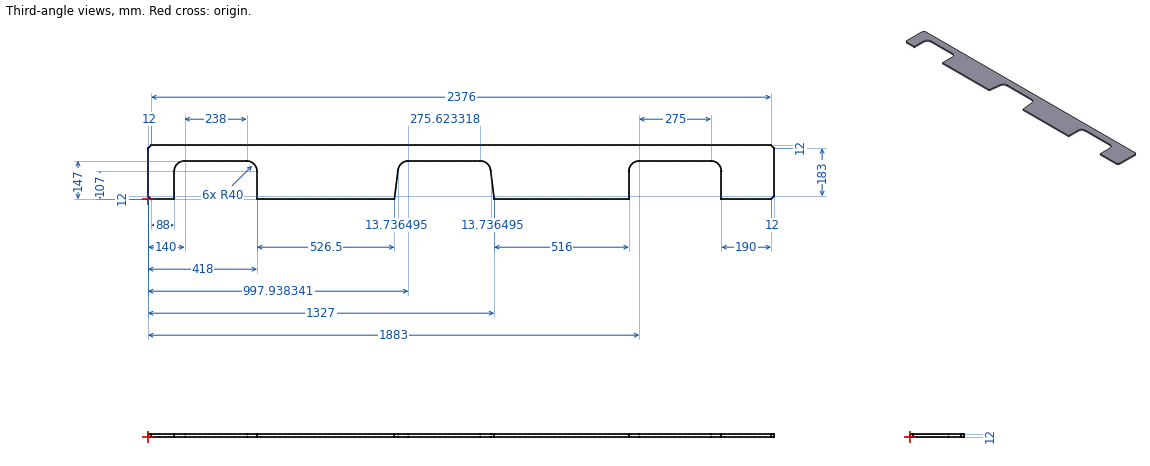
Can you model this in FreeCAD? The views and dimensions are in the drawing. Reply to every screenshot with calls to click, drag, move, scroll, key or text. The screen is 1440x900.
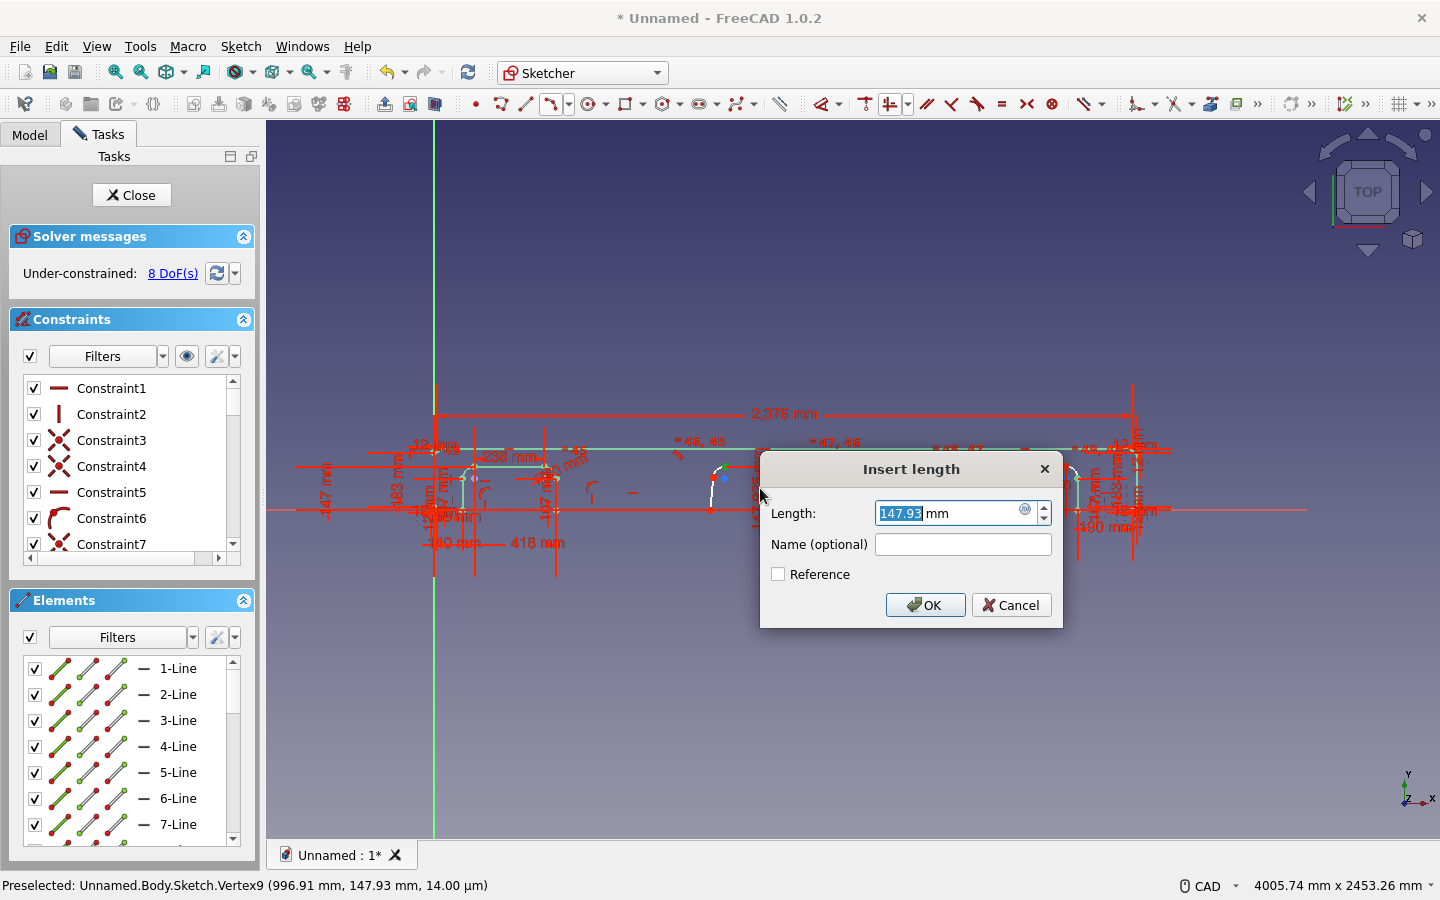
text(147)
key(Return)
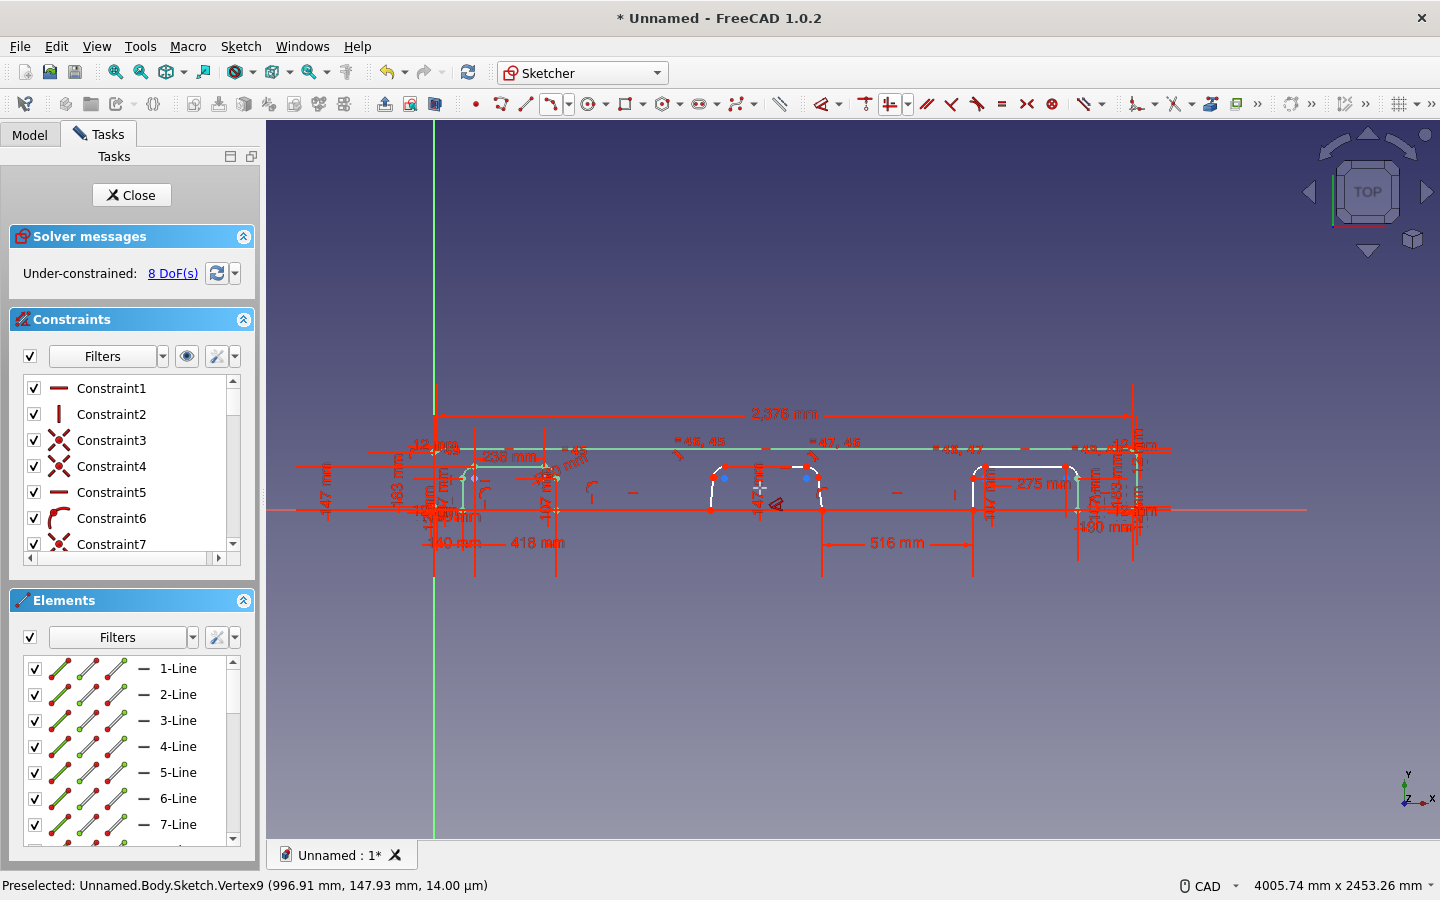
click(985, 467)
click(400, 498)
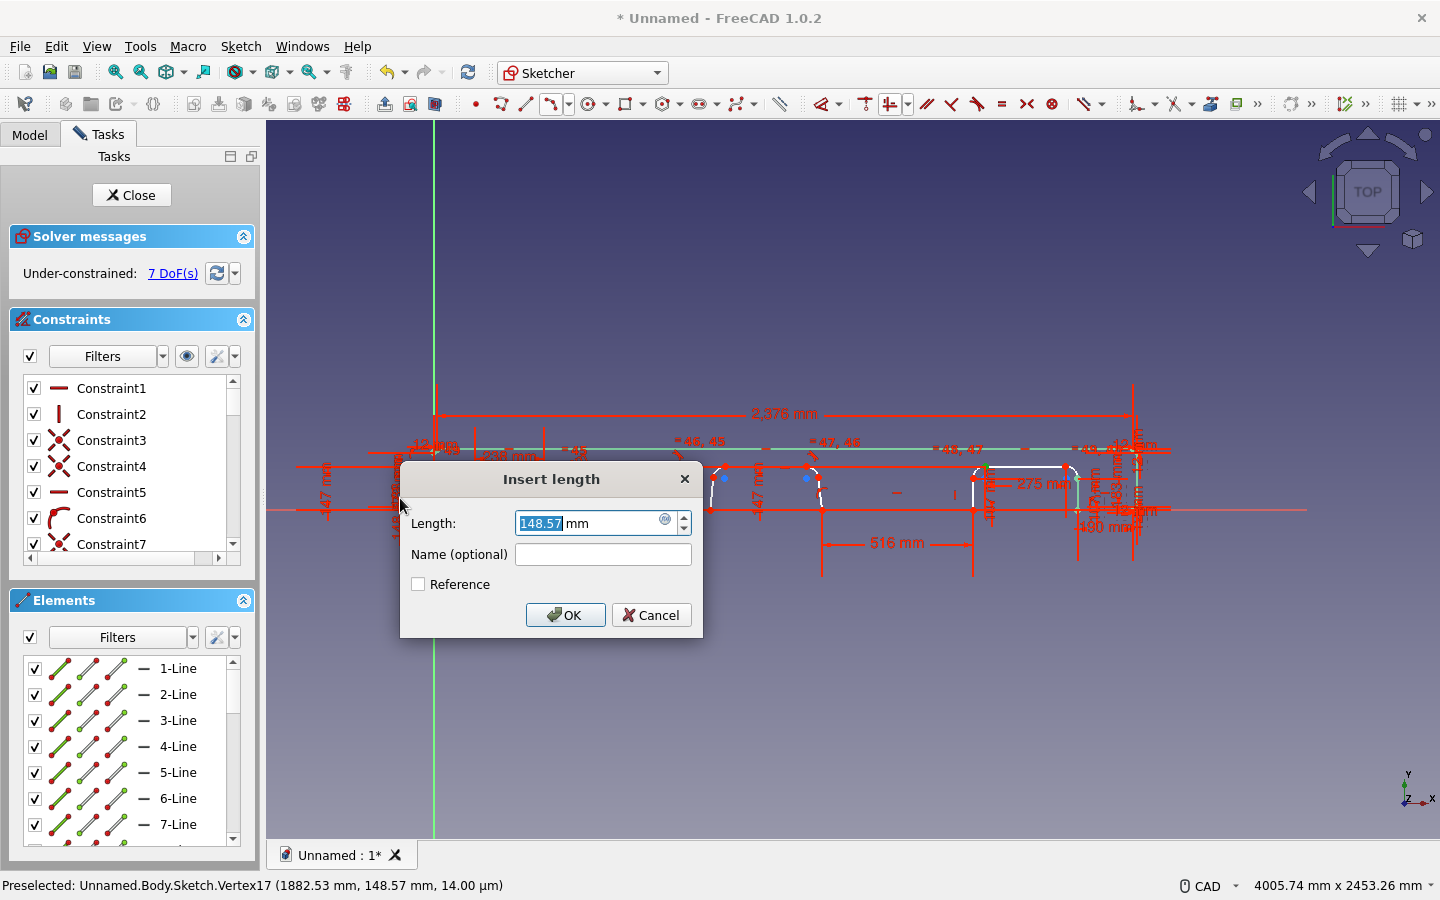
text(147)
key(Return)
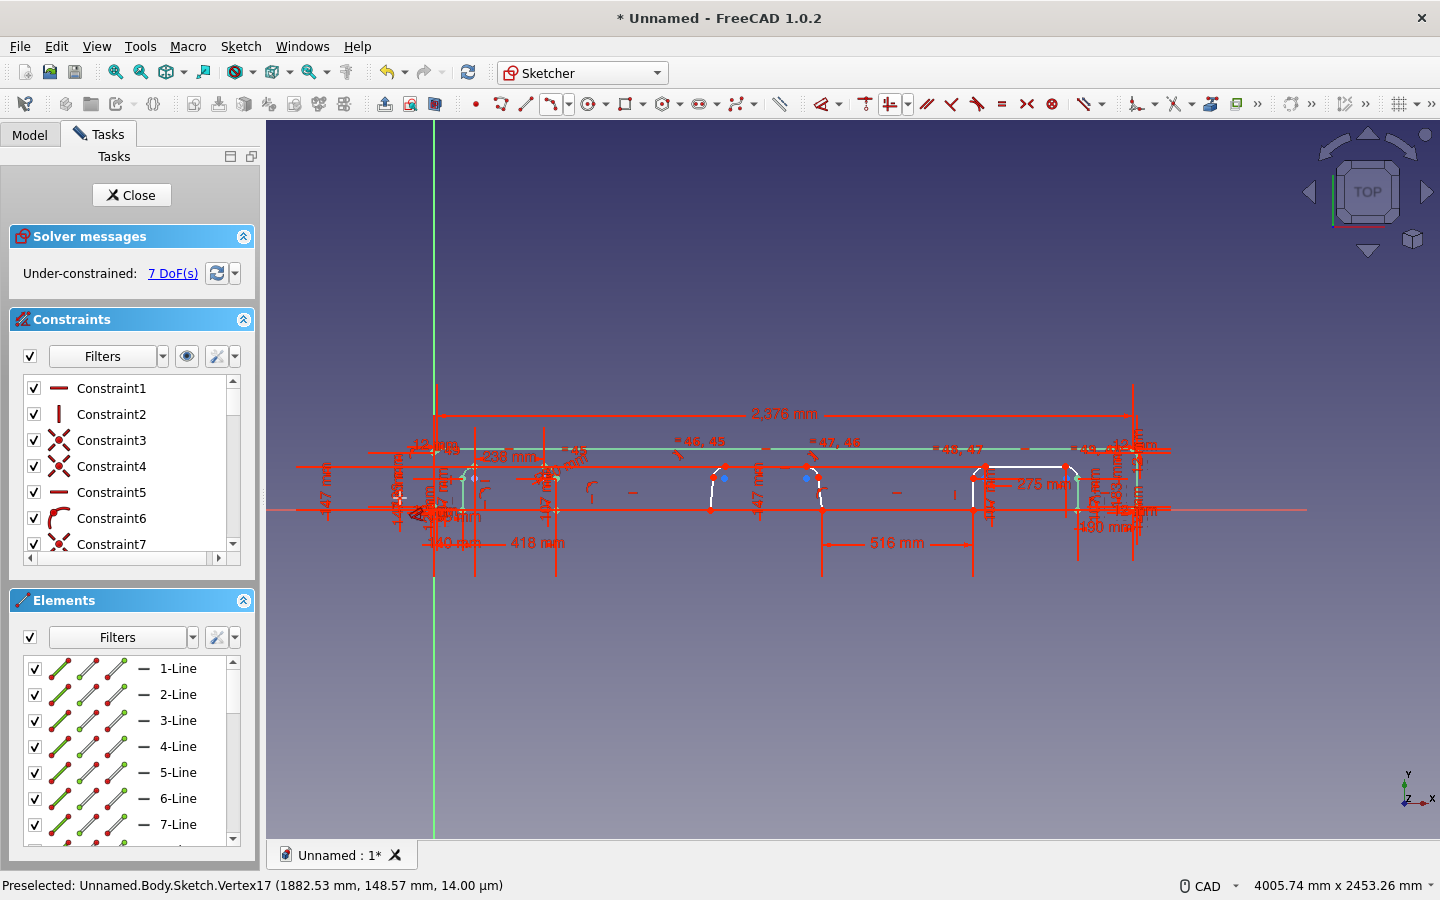
click(602, 510)
click(633, 544)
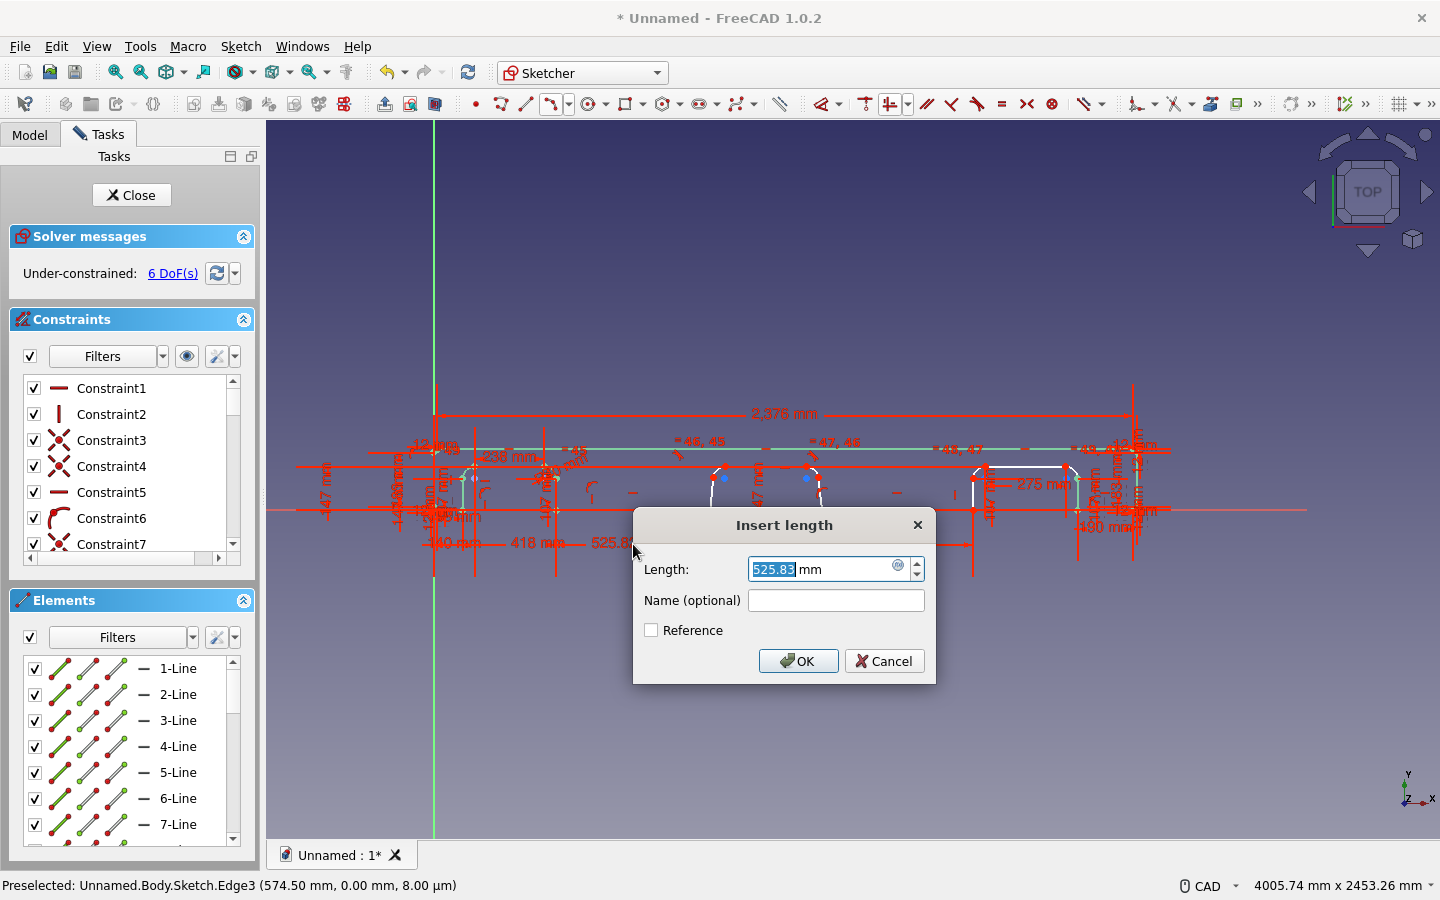
text(526.5)
key(Return)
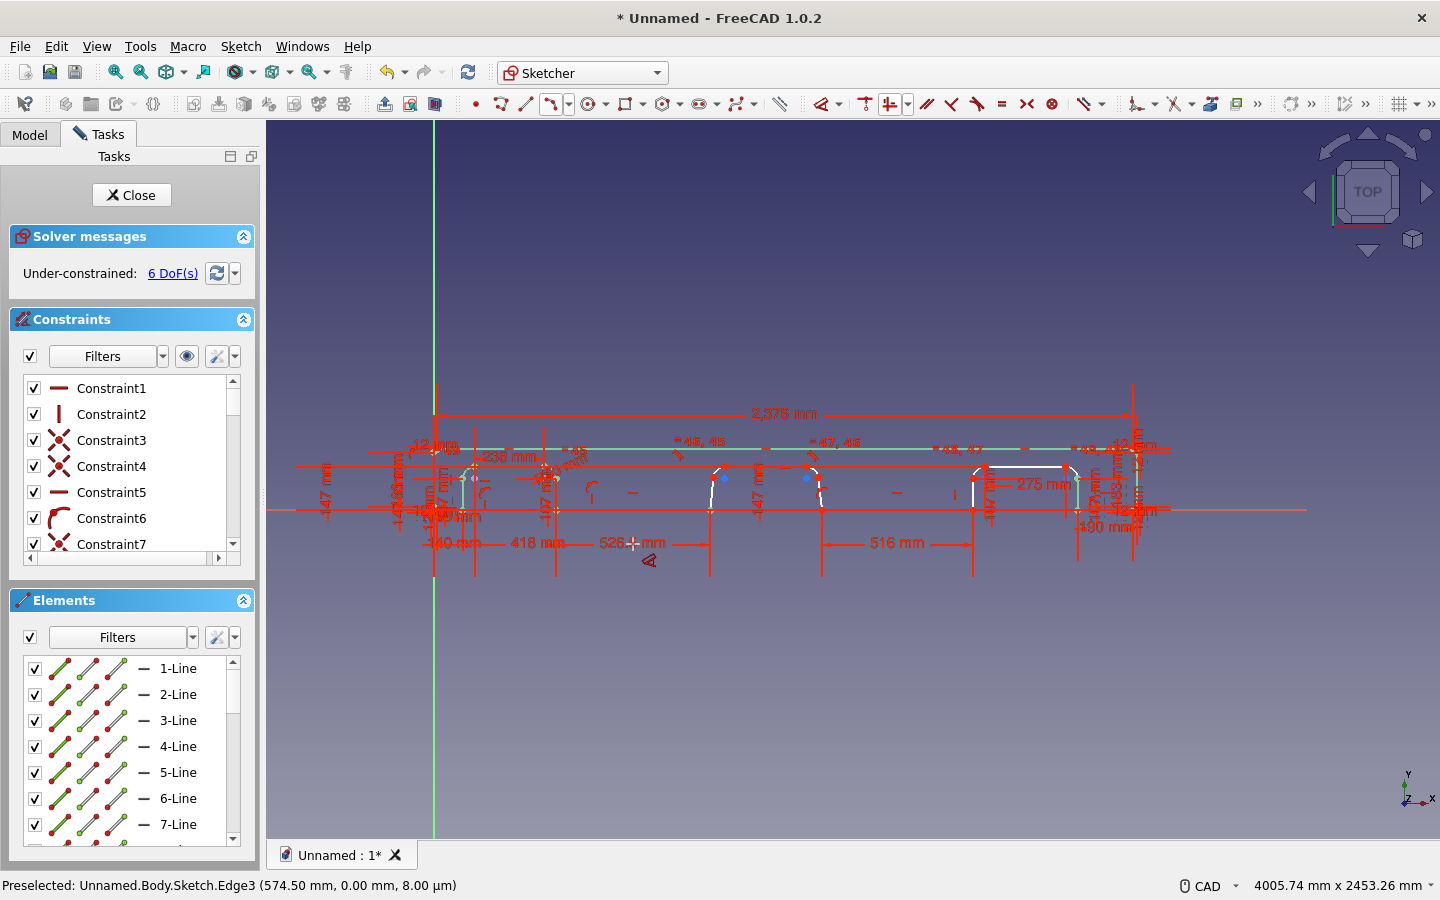
click(822, 510)
click(717, 544)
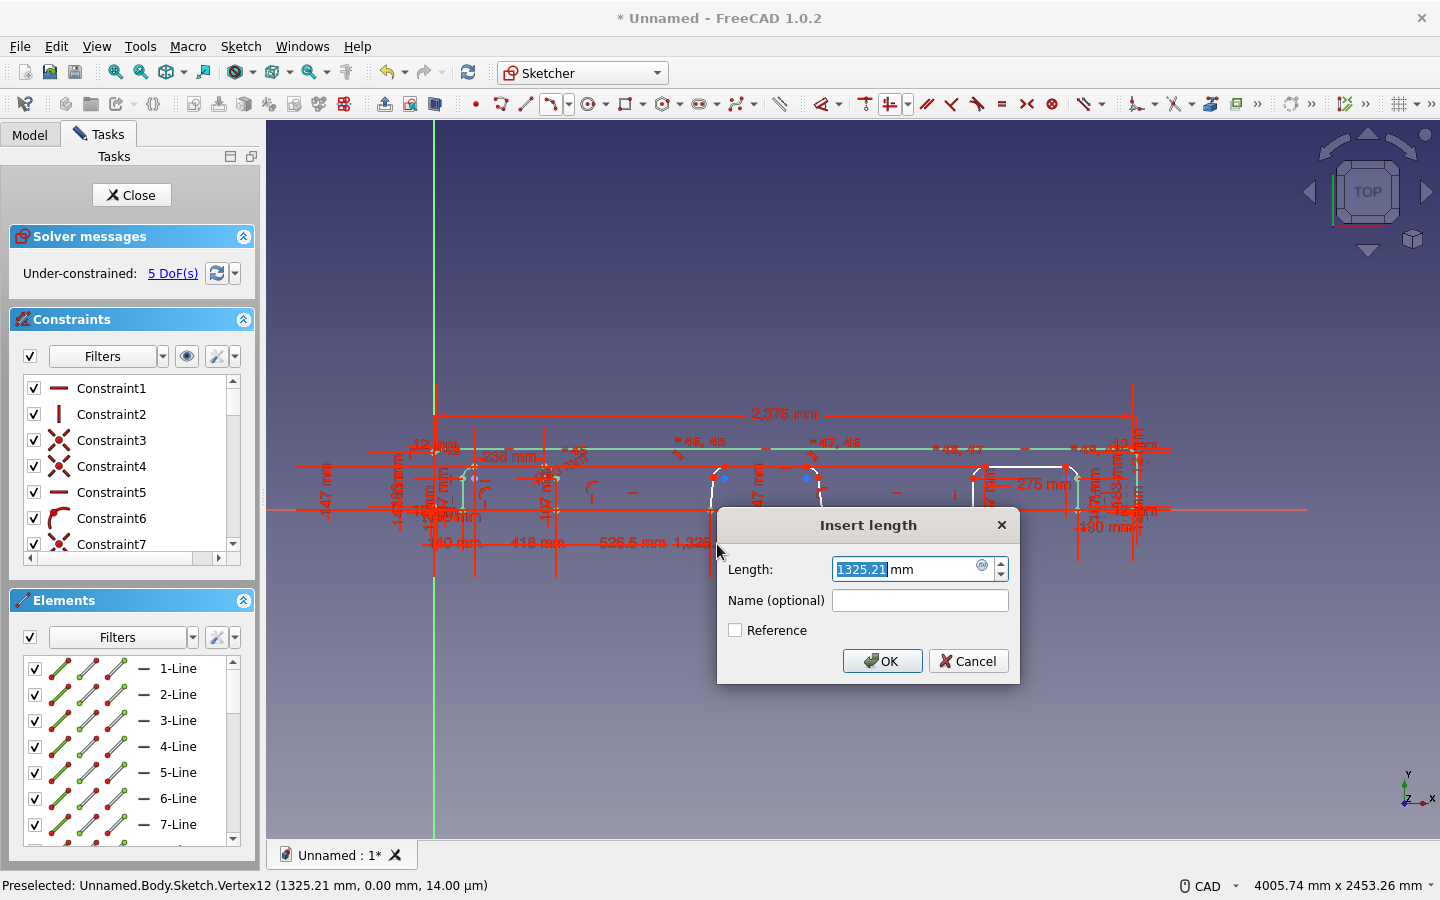
text(1327)
key(Return)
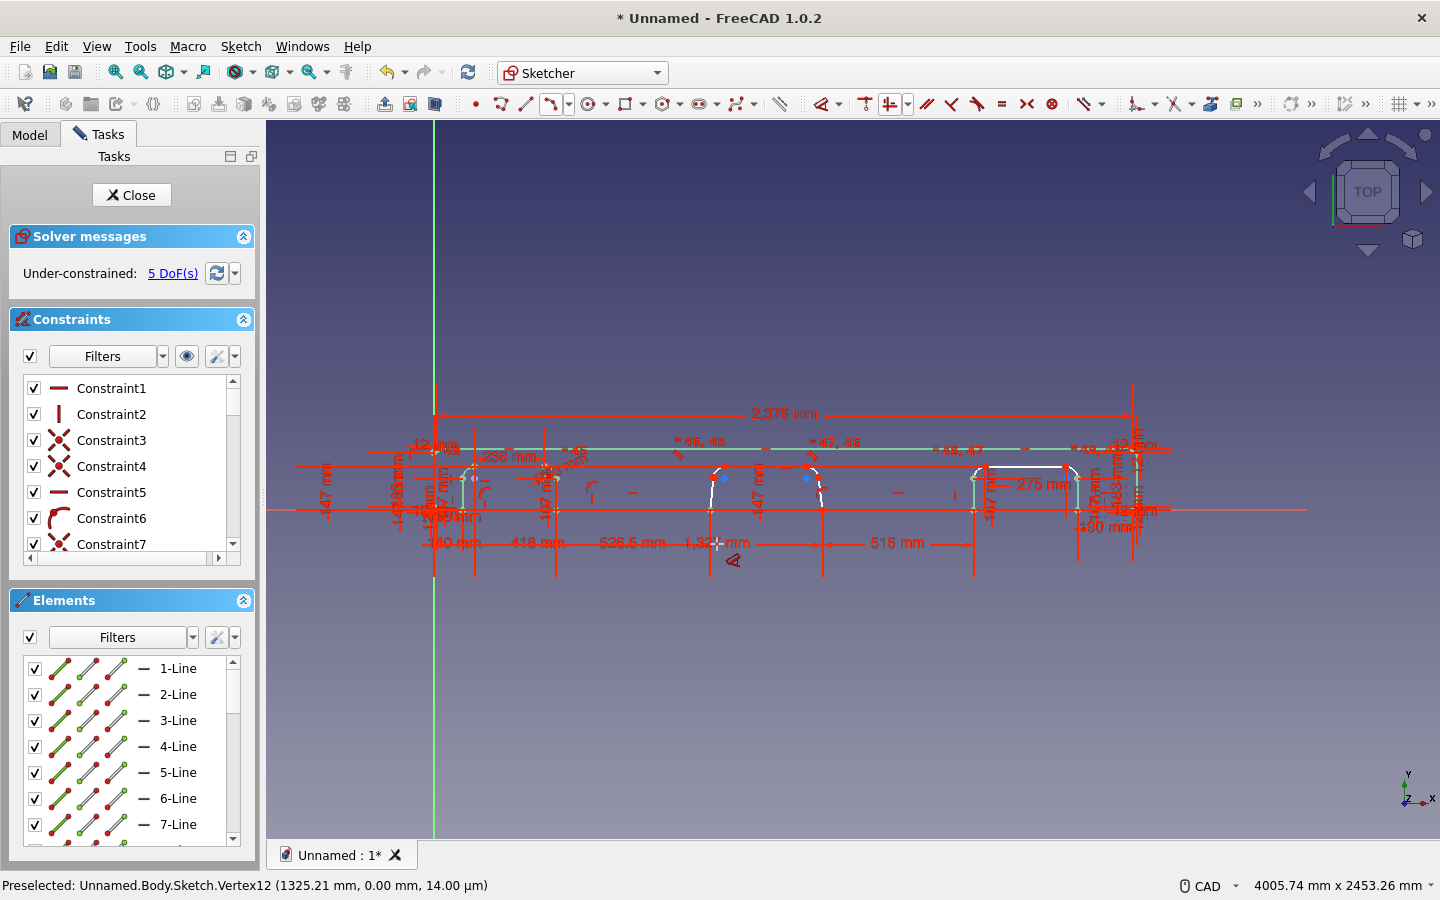
click(985, 467)
click(709, 433)